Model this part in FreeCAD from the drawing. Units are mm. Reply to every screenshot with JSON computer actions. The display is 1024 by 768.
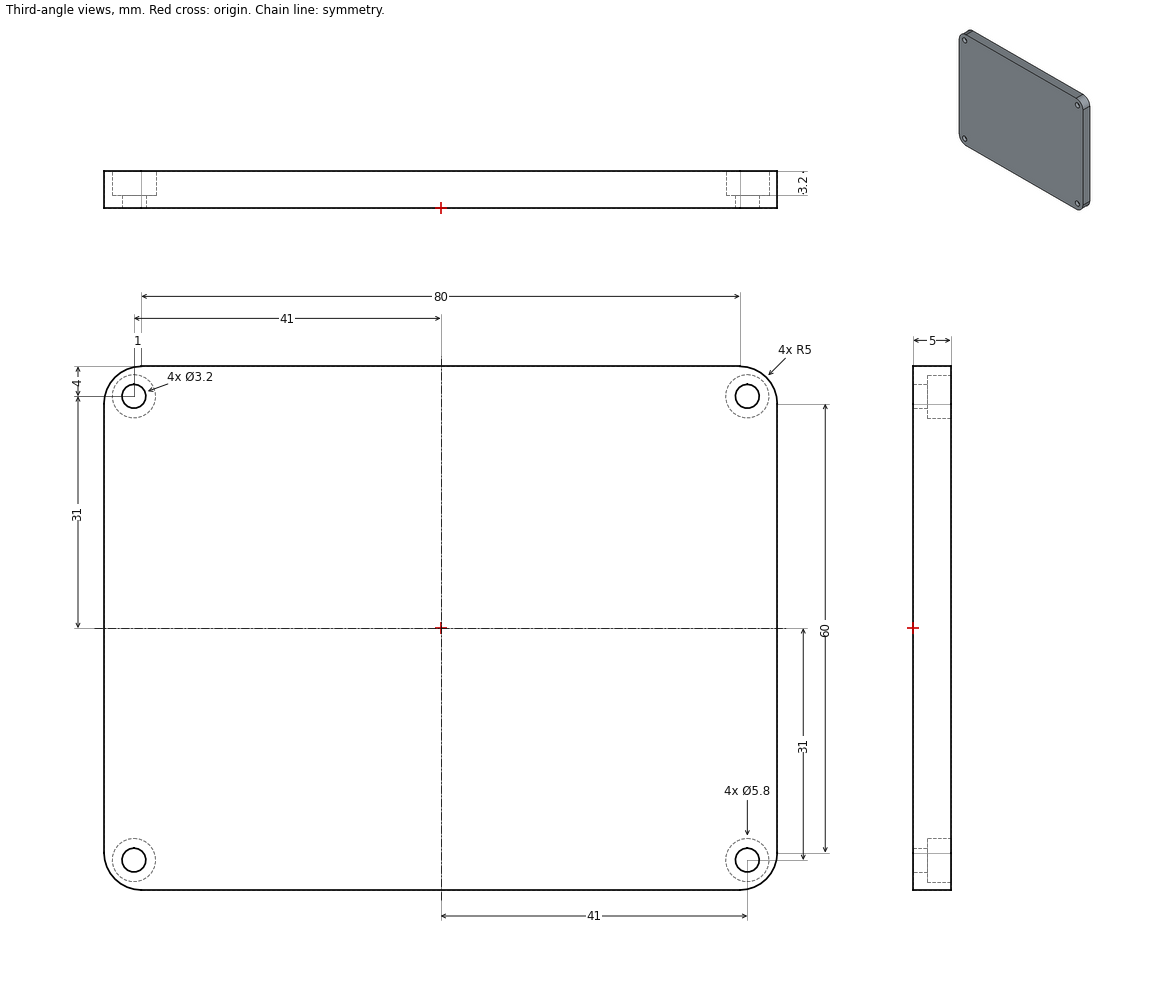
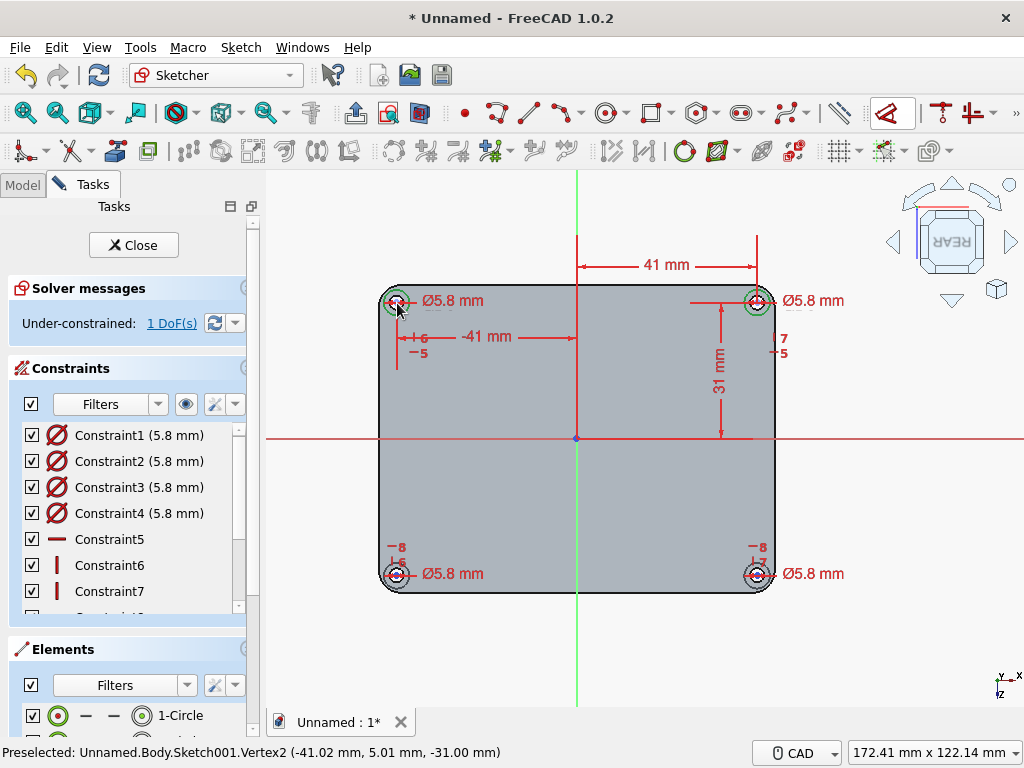
{"action": "left_click", "coordinate": [397, 576]}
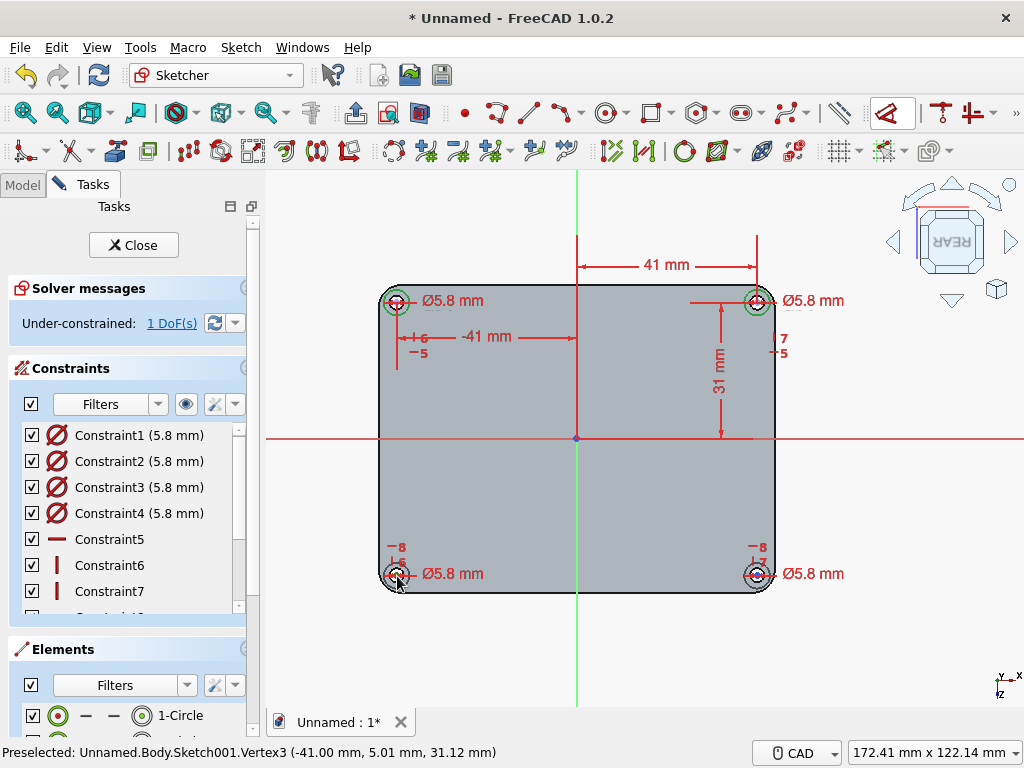
{"action": "key", "text": "i"}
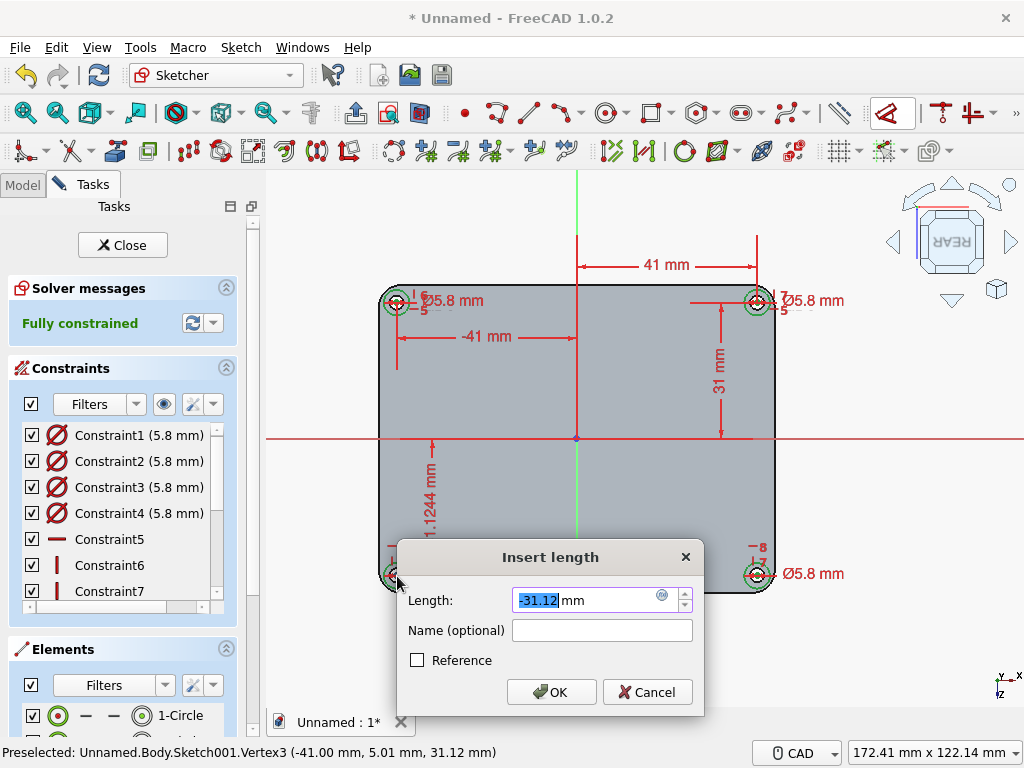
{"action": "type", "text": "-31"}
{"action": "key", "text": "Return"}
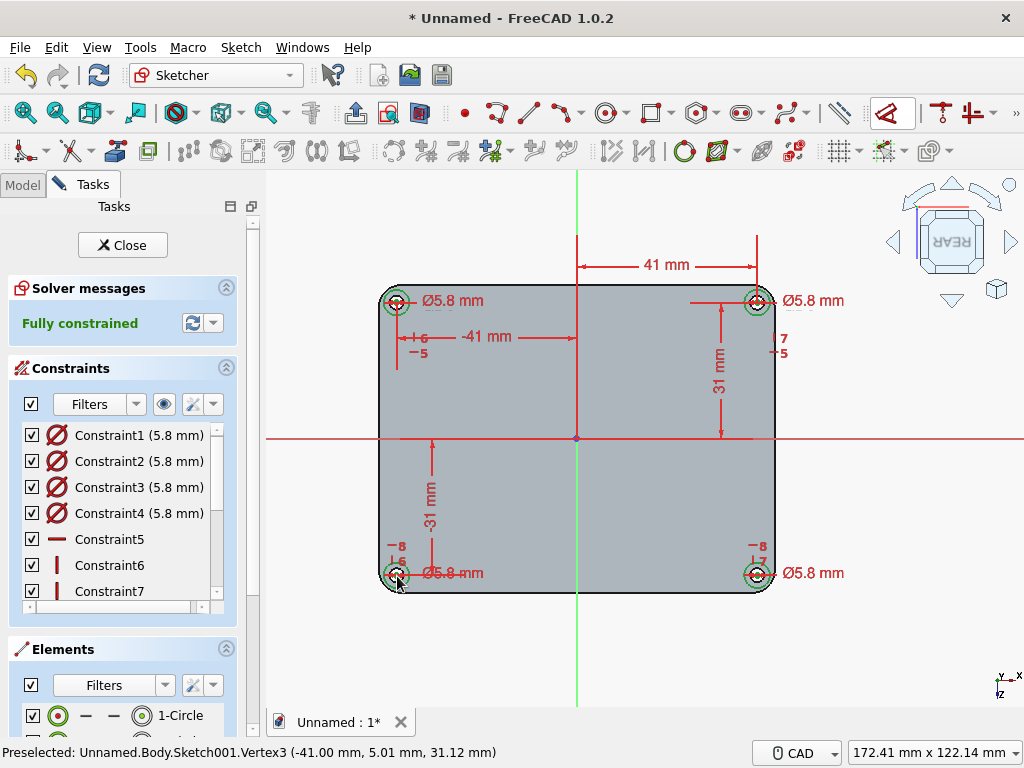
{"action": "left_click", "coordinate": [123, 245]}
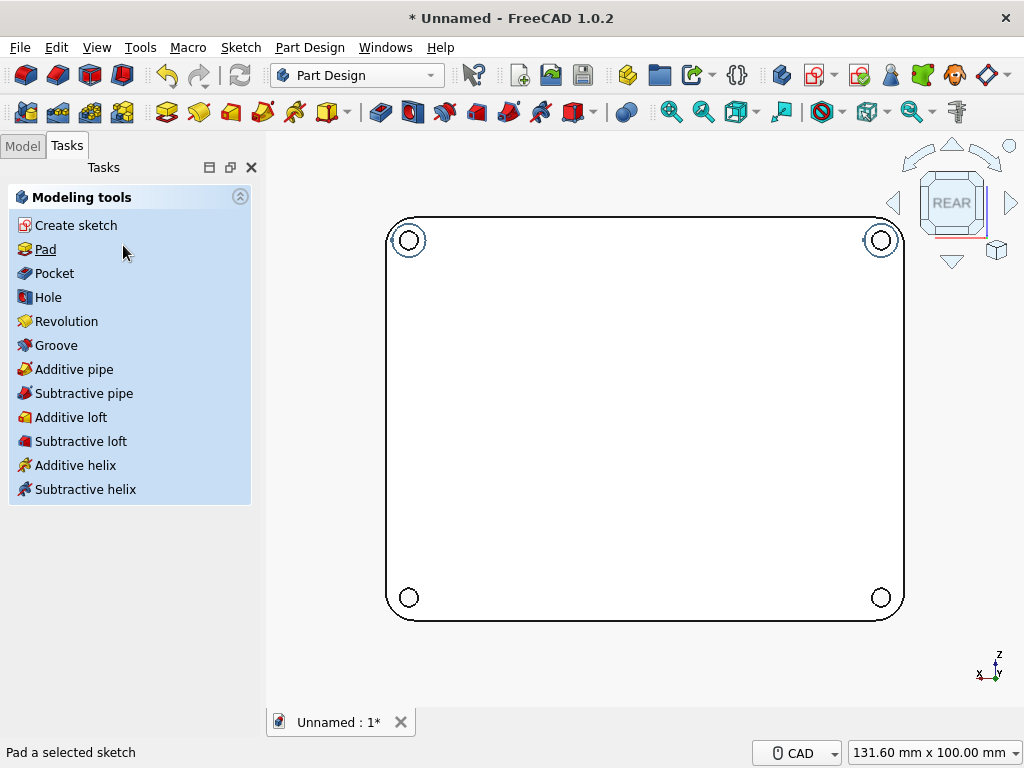
{"action": "left_click", "coordinate": [382, 112]}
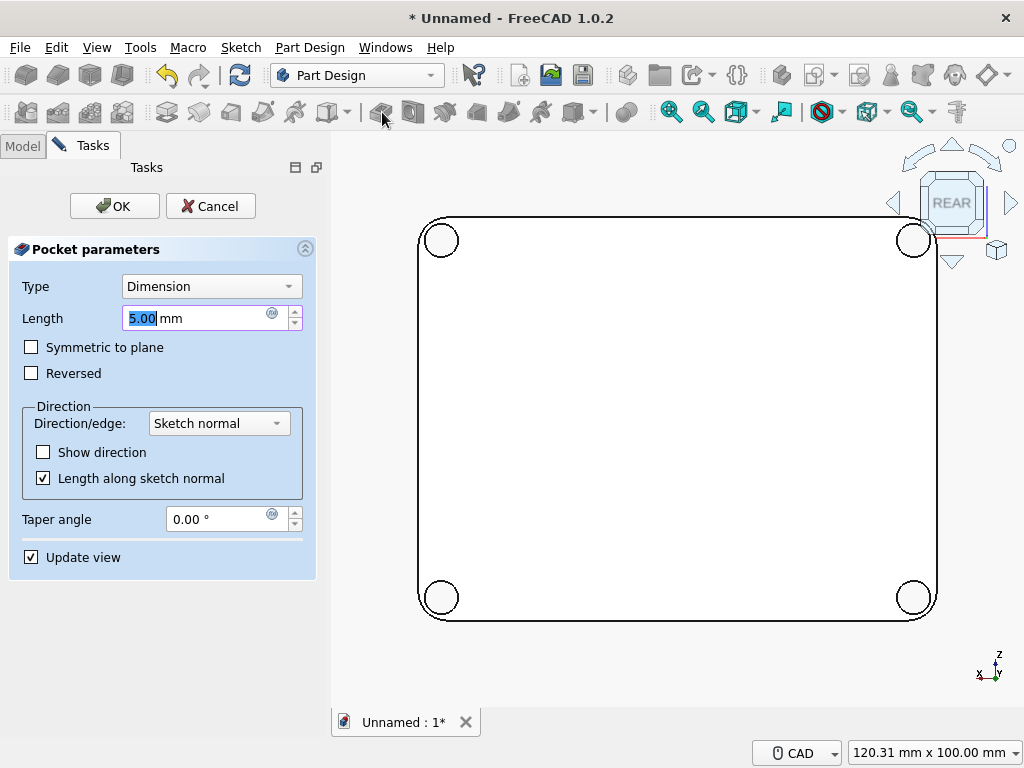
{"action": "type", "text": "3.2"}
{"action": "key", "text": "Tab"}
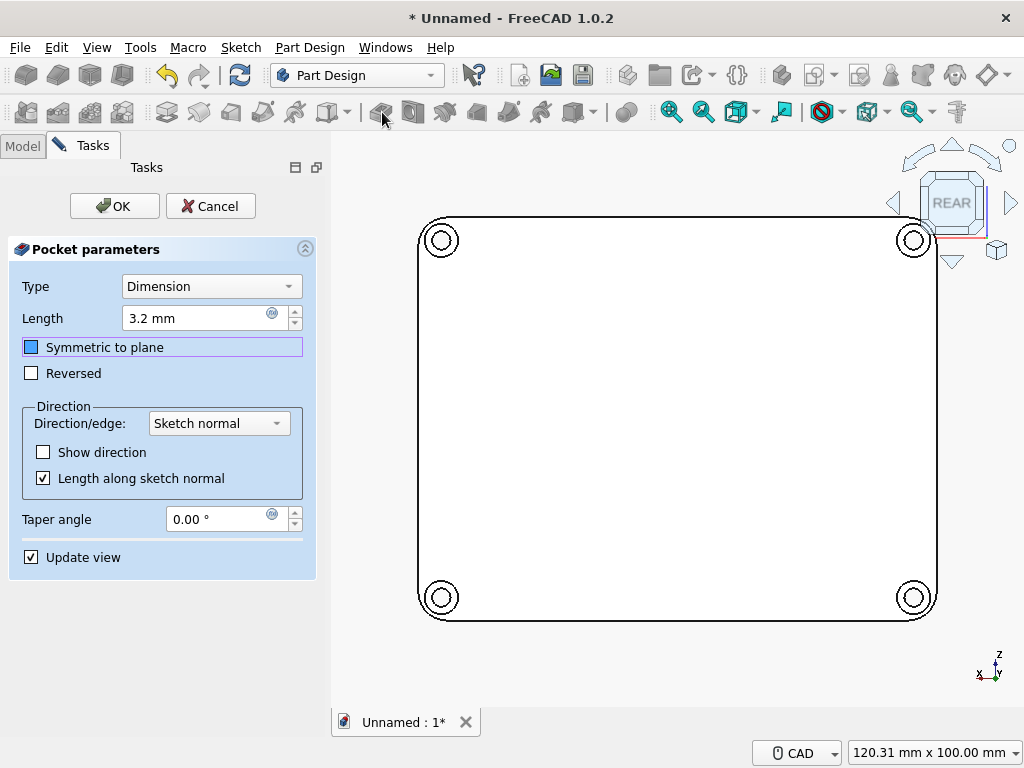
{"action": "left_click", "coordinate": [115, 206]}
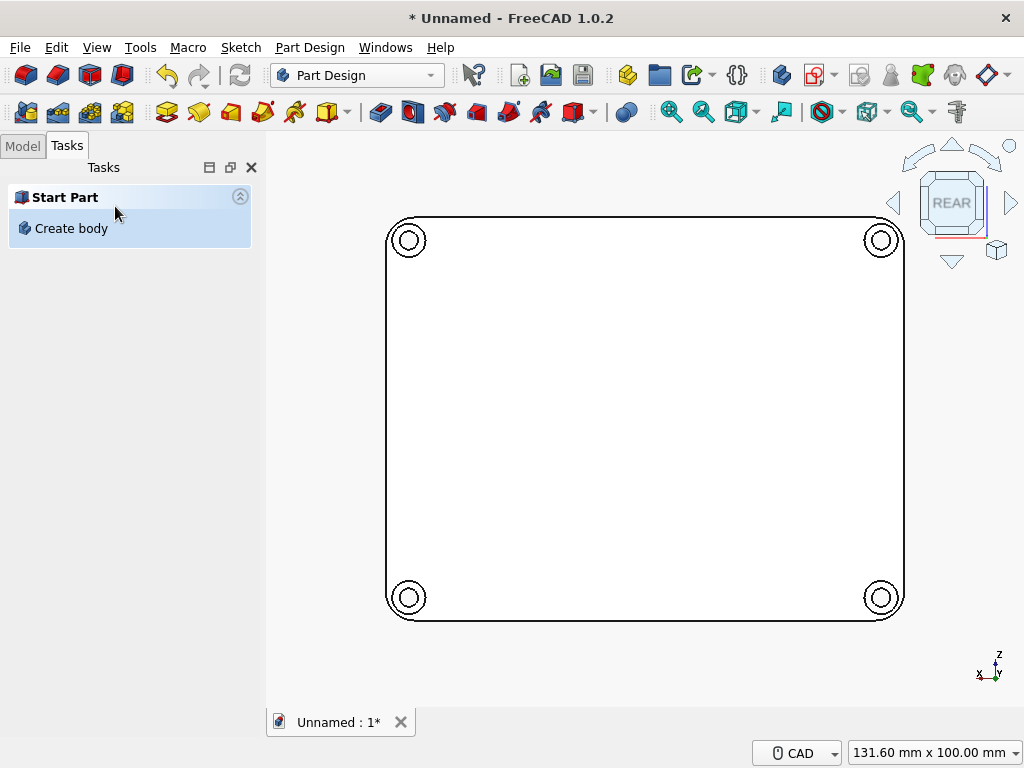
{"action": "key", "text": "0"}